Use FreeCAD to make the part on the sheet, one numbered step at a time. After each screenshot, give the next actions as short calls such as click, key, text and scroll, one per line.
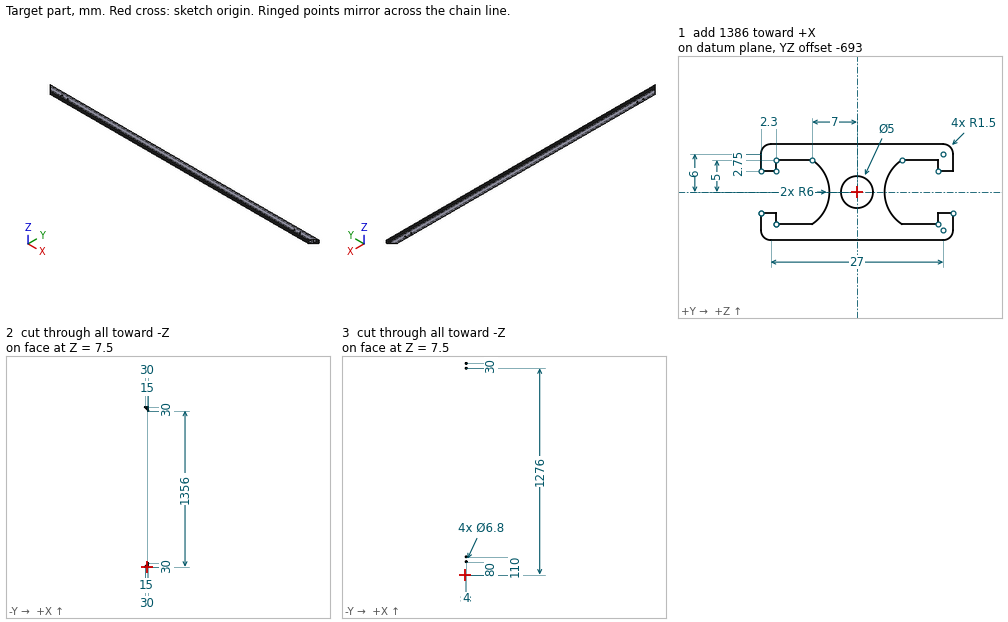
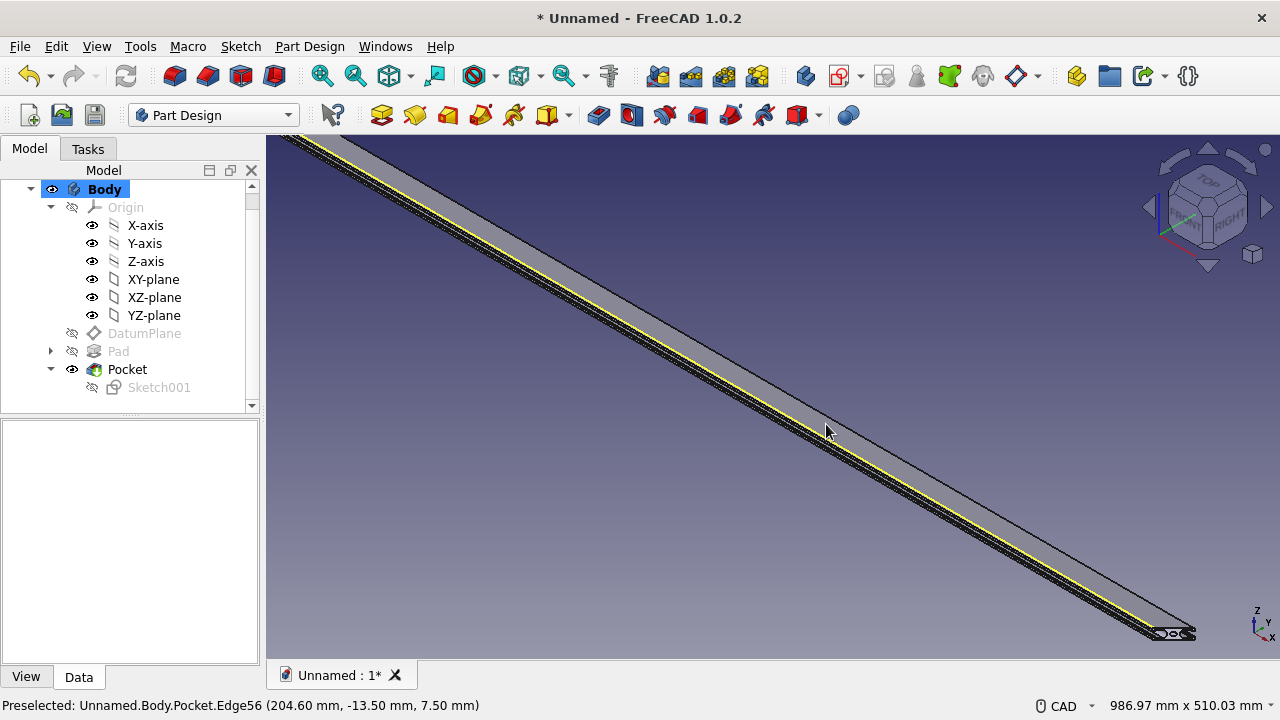
click(825, 425)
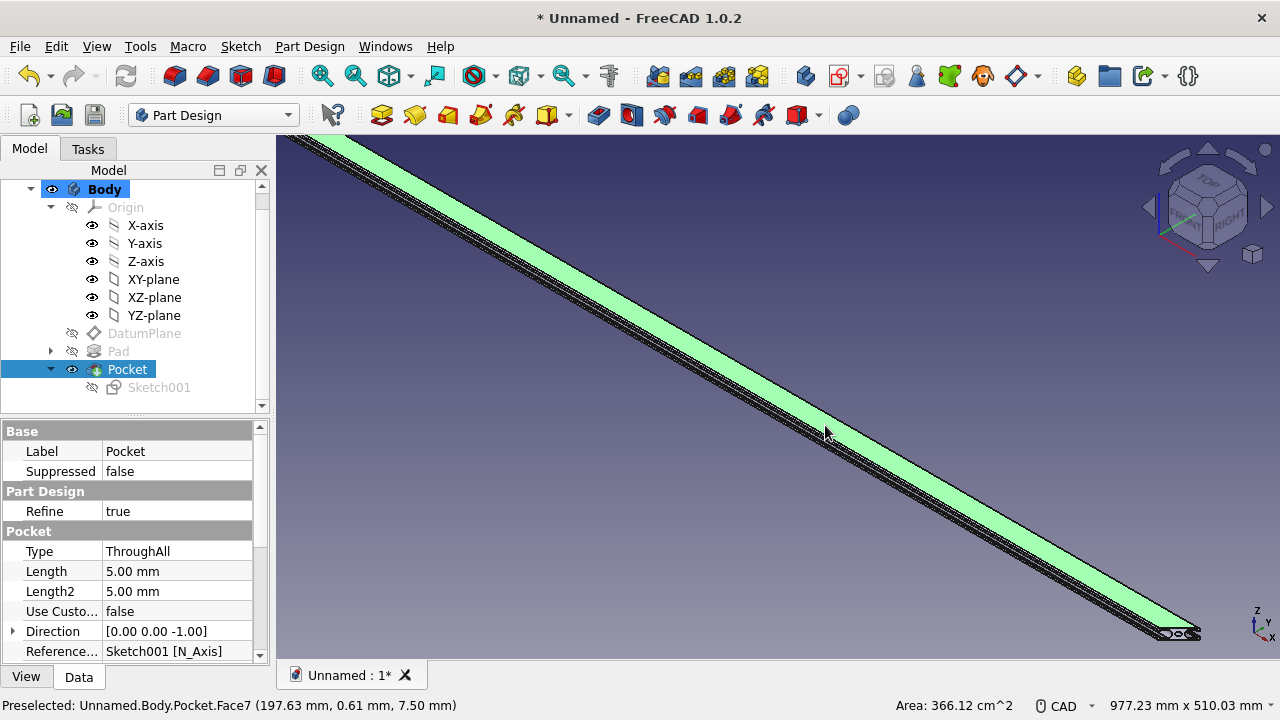
click(838, 76)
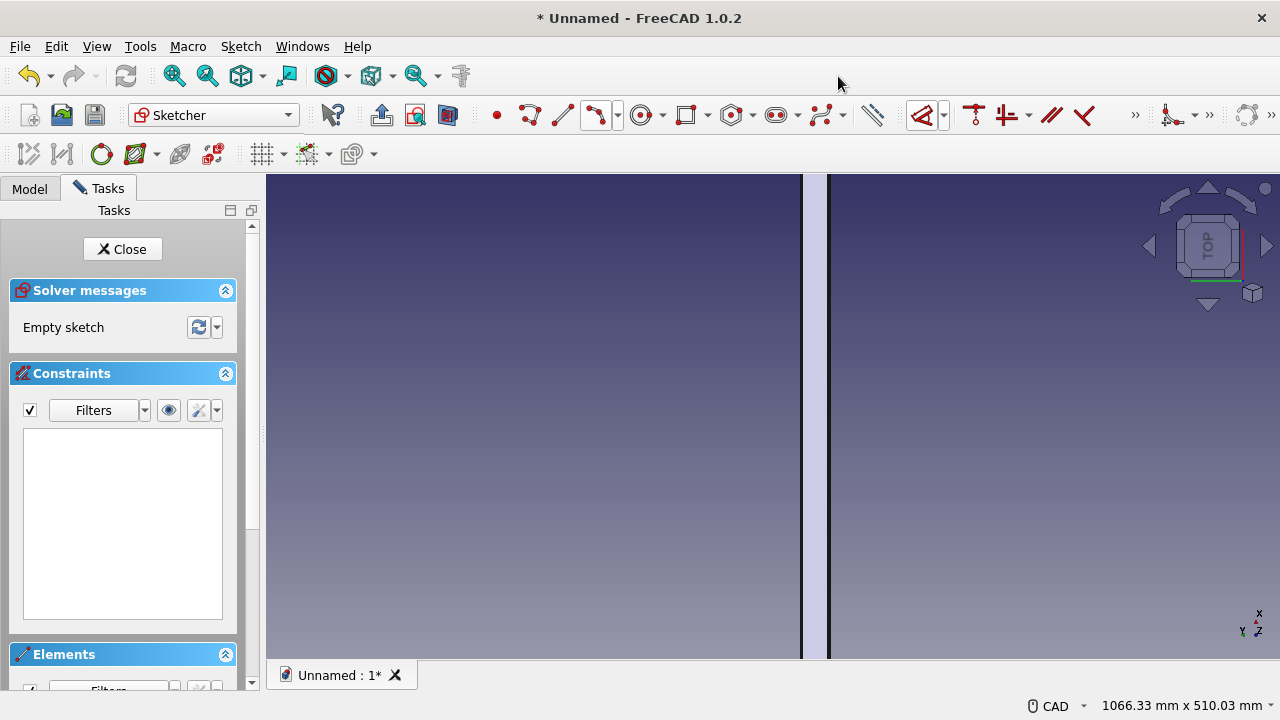
scroll(667, 379, down, 7)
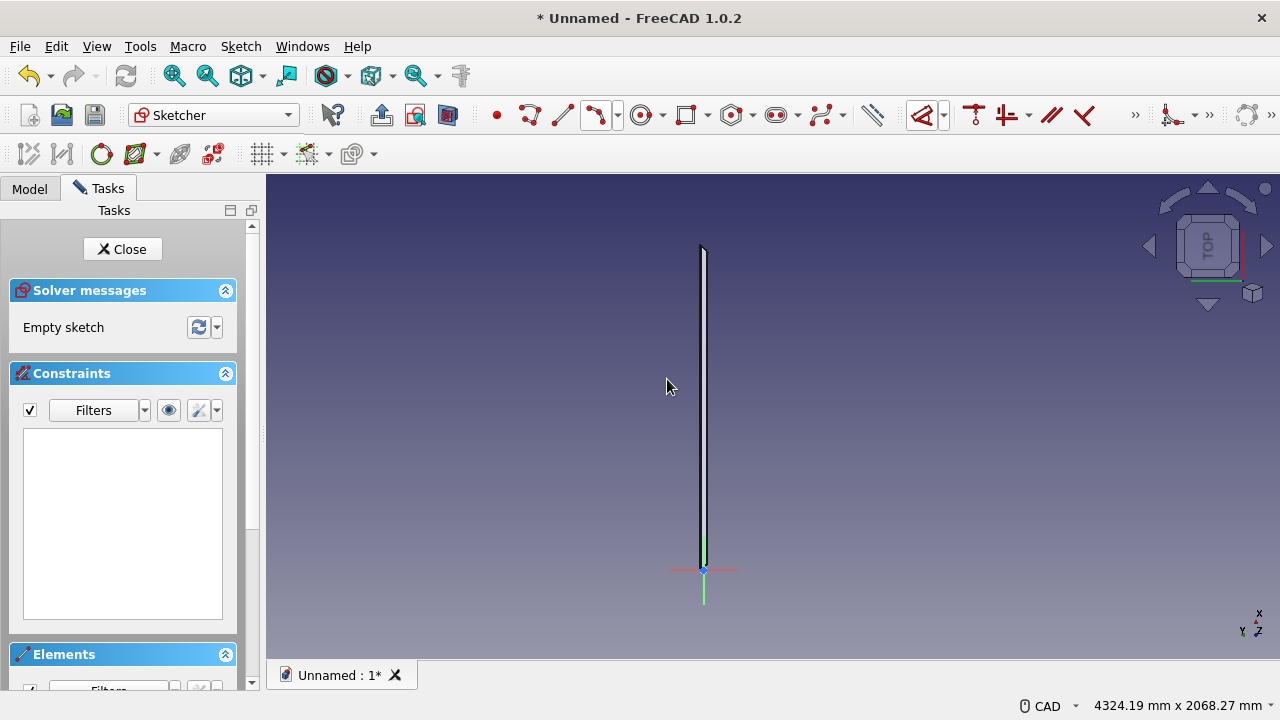
click(640, 116)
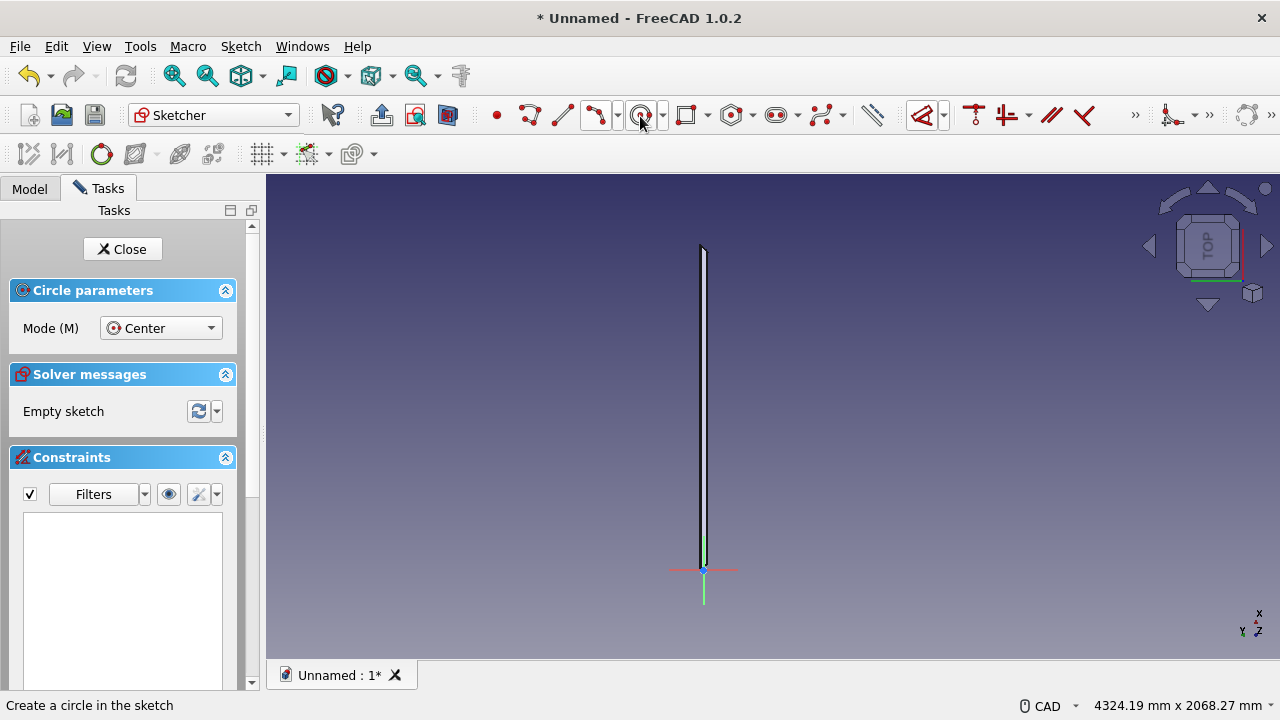
scroll(705, 552, up, 17)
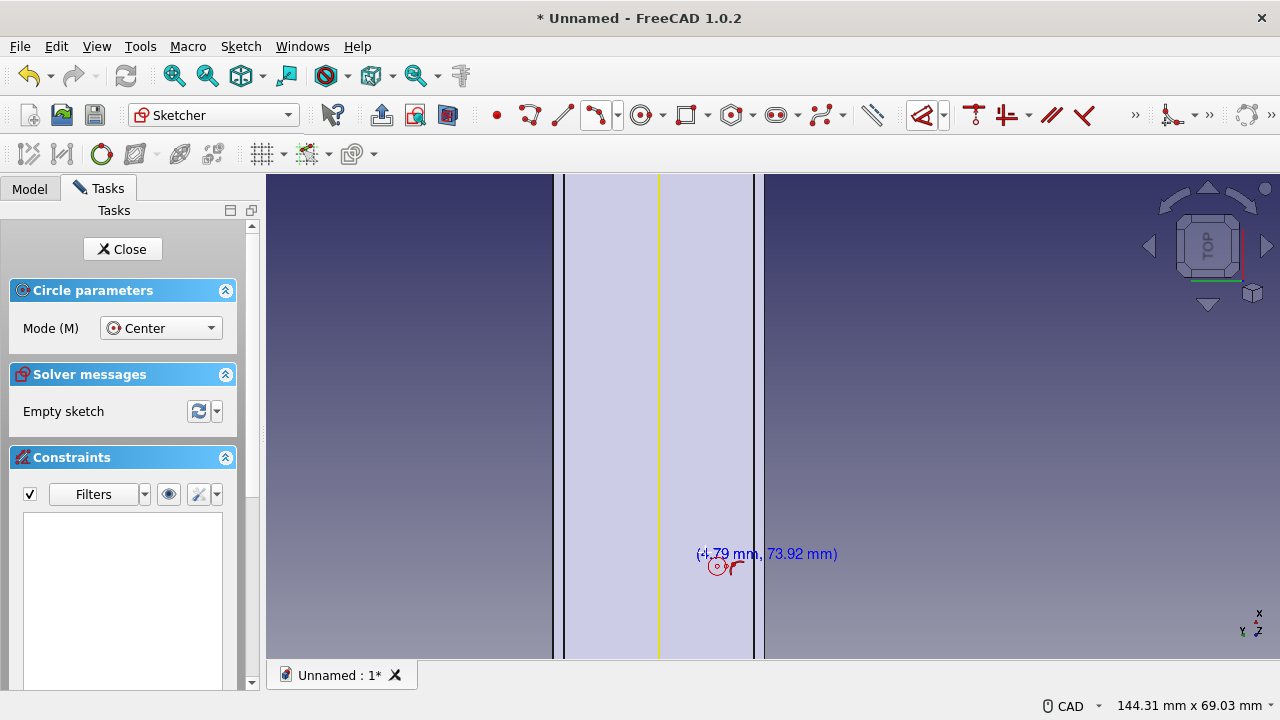
click(687, 517)
click(704, 500)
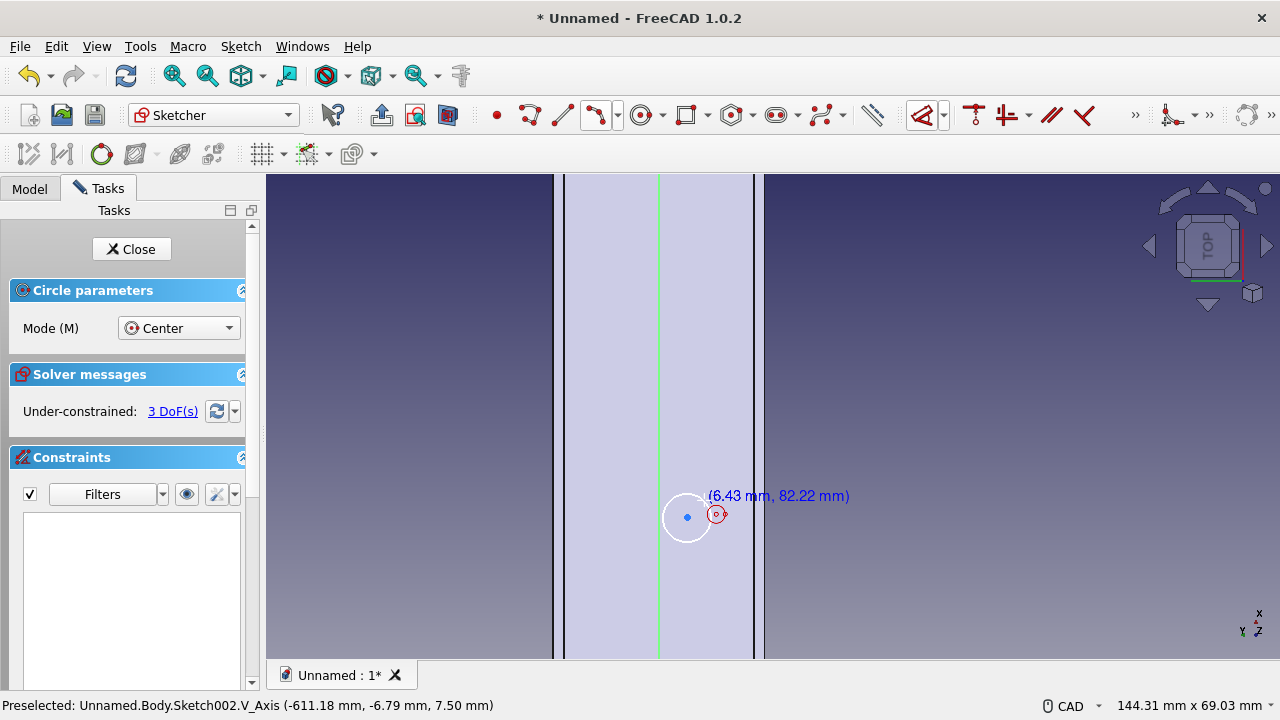
click(687, 306)
click(704, 289)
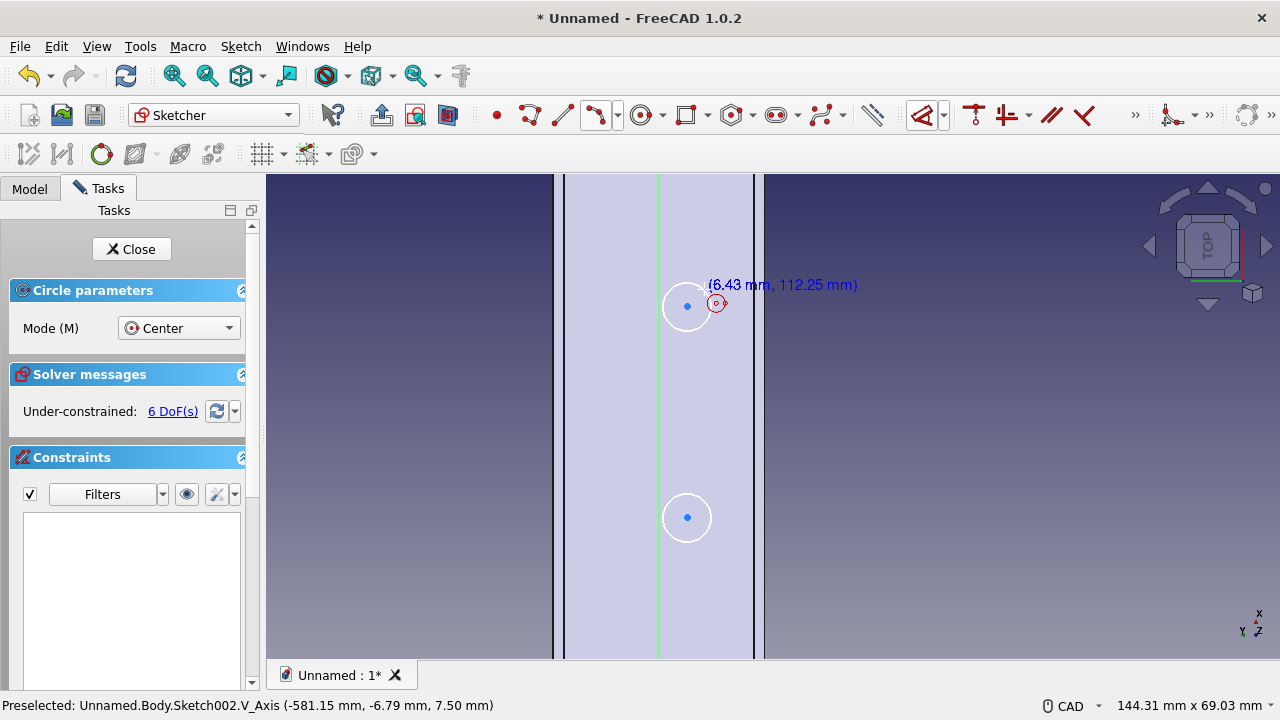
scroll(705, 584, down, 16)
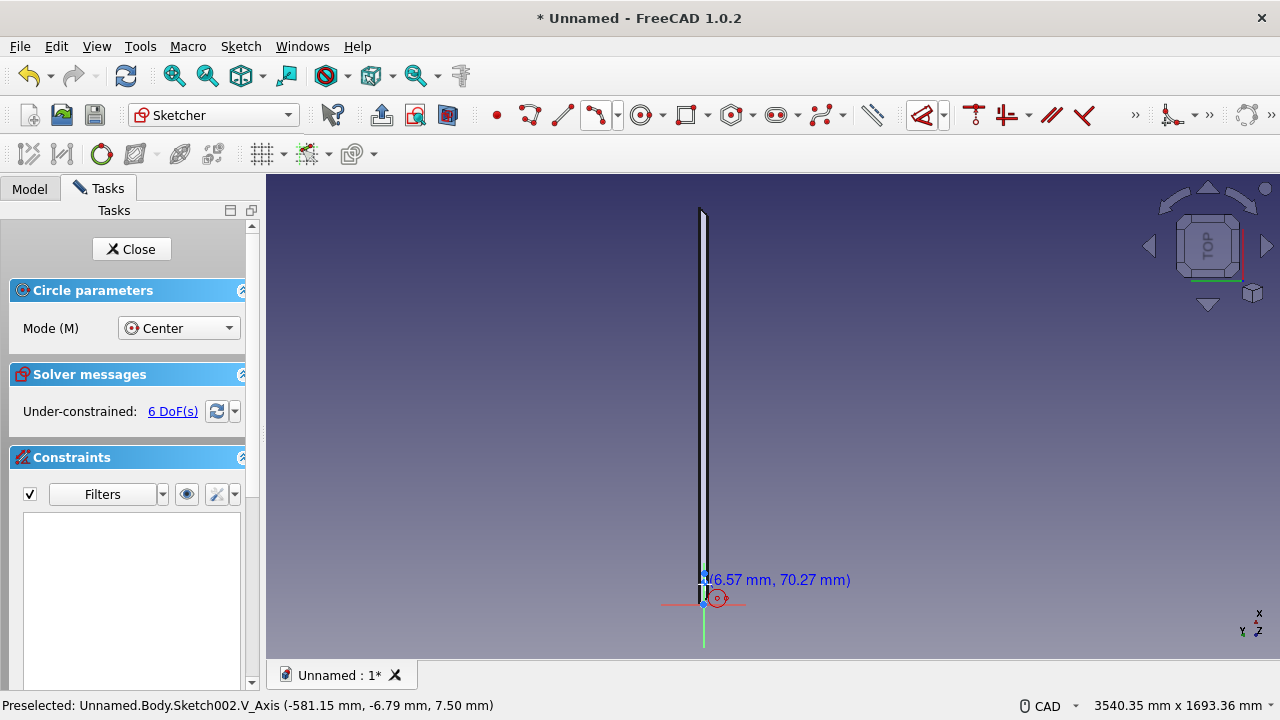
scroll(705, 240, up, 16)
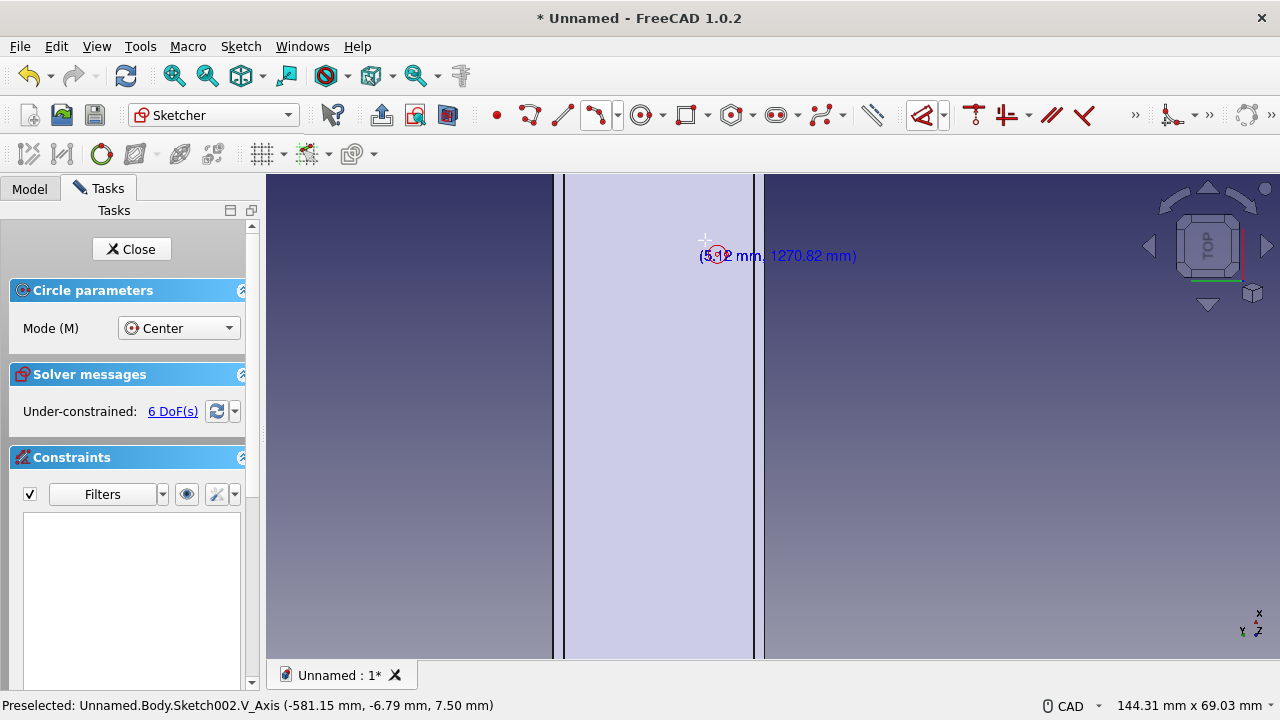
click(687, 225)
click(704, 208)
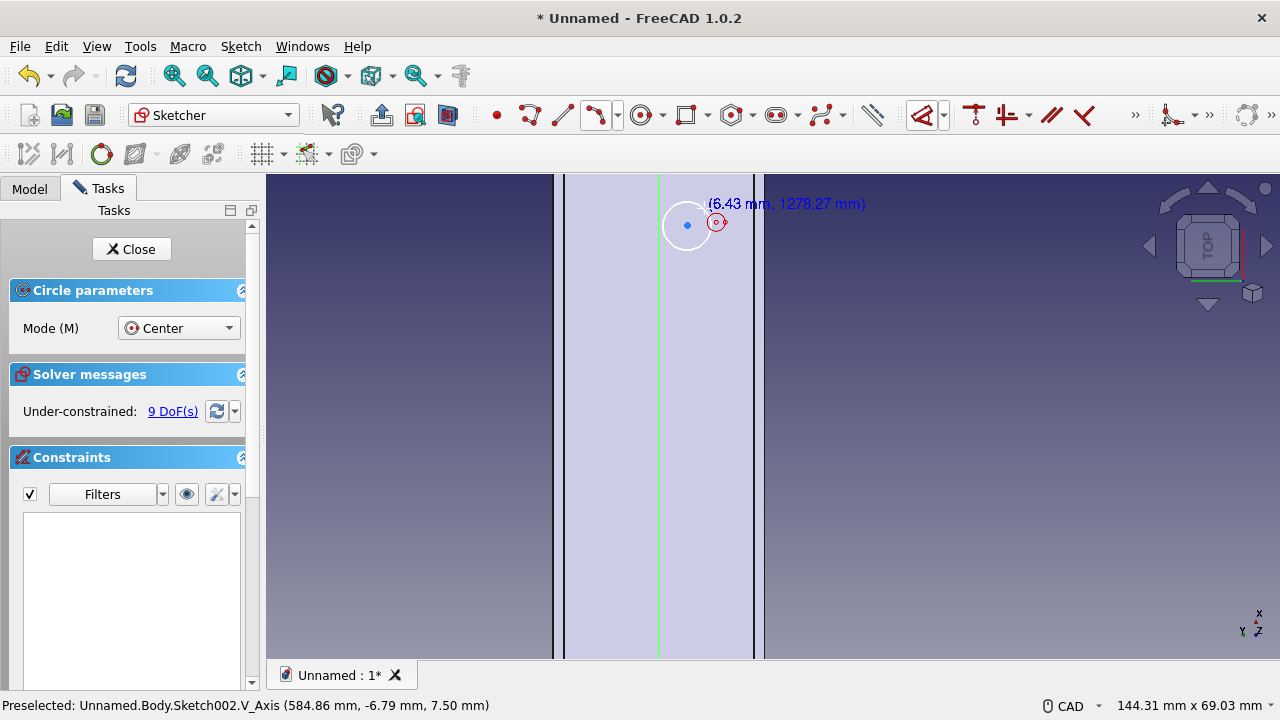
scroll(705, 239, down, 16)